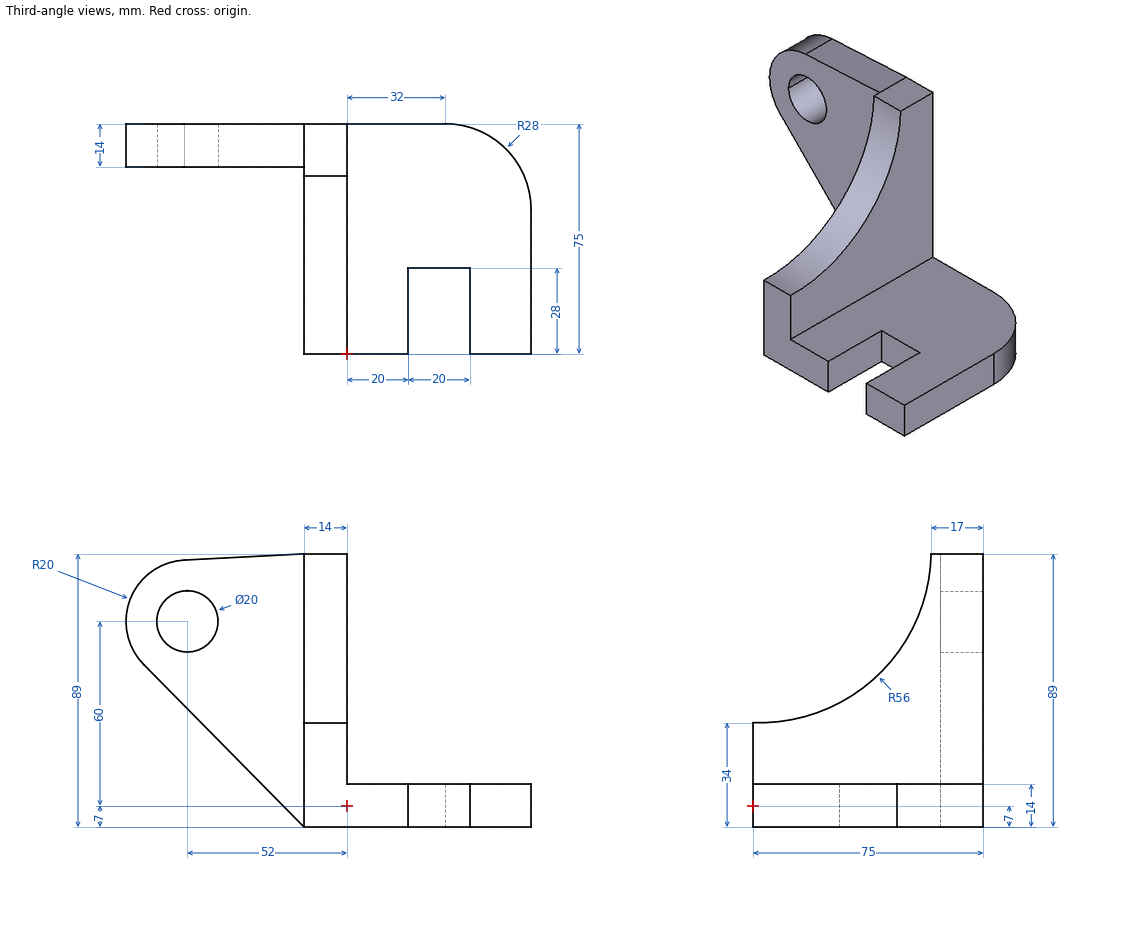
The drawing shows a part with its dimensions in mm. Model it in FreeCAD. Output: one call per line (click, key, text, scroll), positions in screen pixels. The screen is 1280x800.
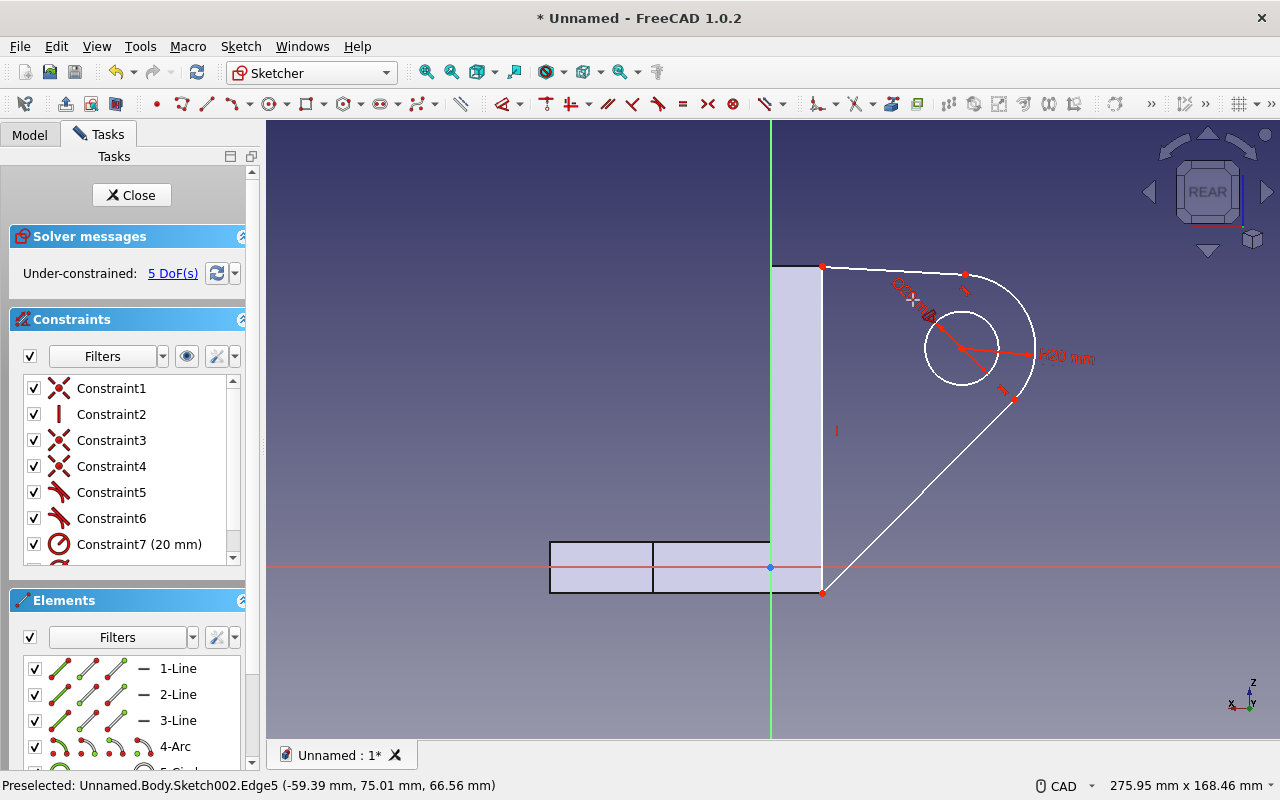
click(822, 365)
click(788, 430)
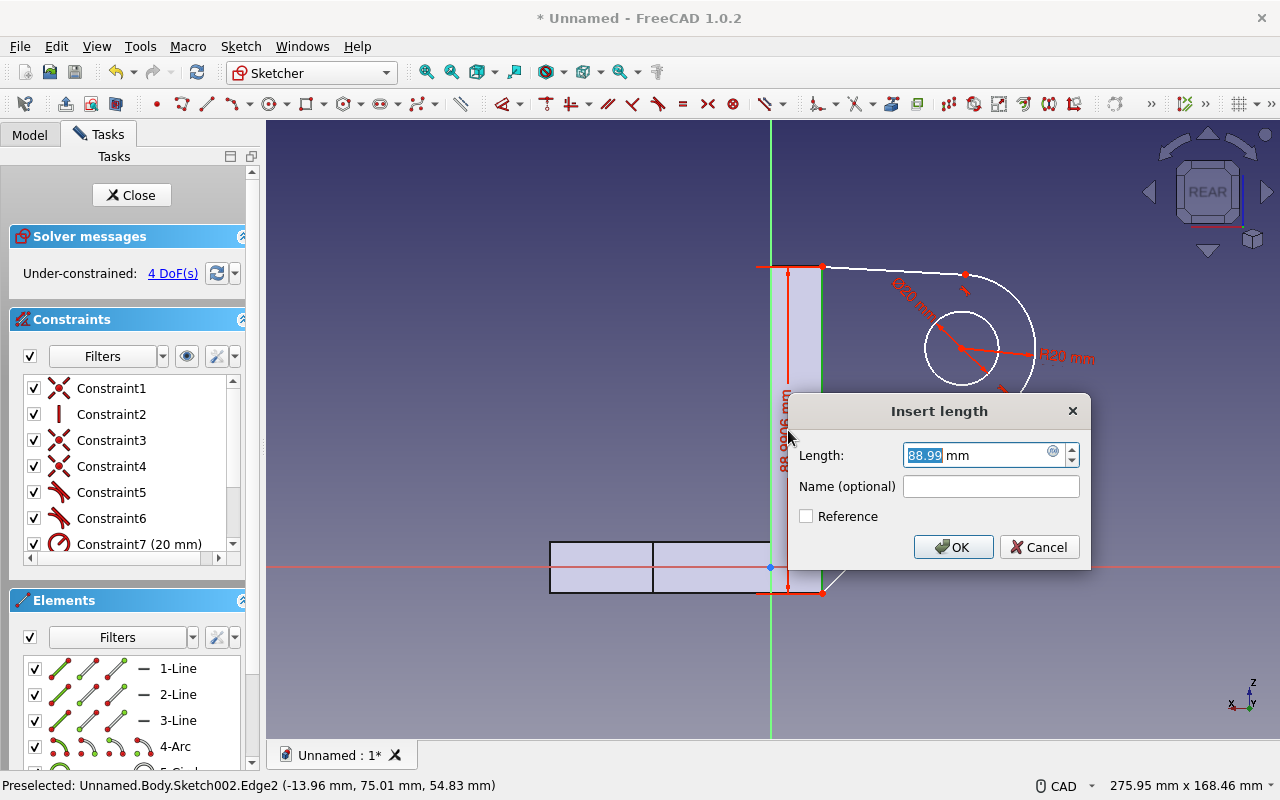
text(89)
key(Return)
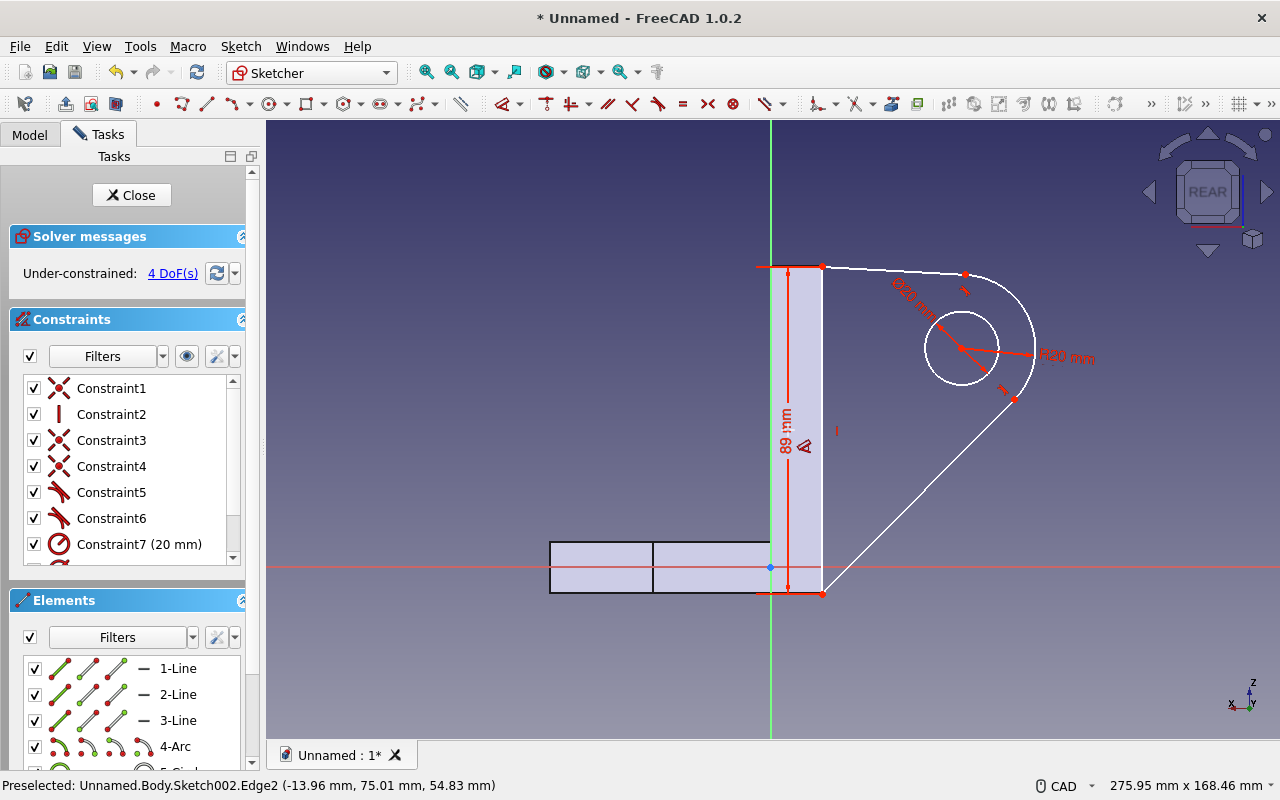
scroll(822, 594, up, 3)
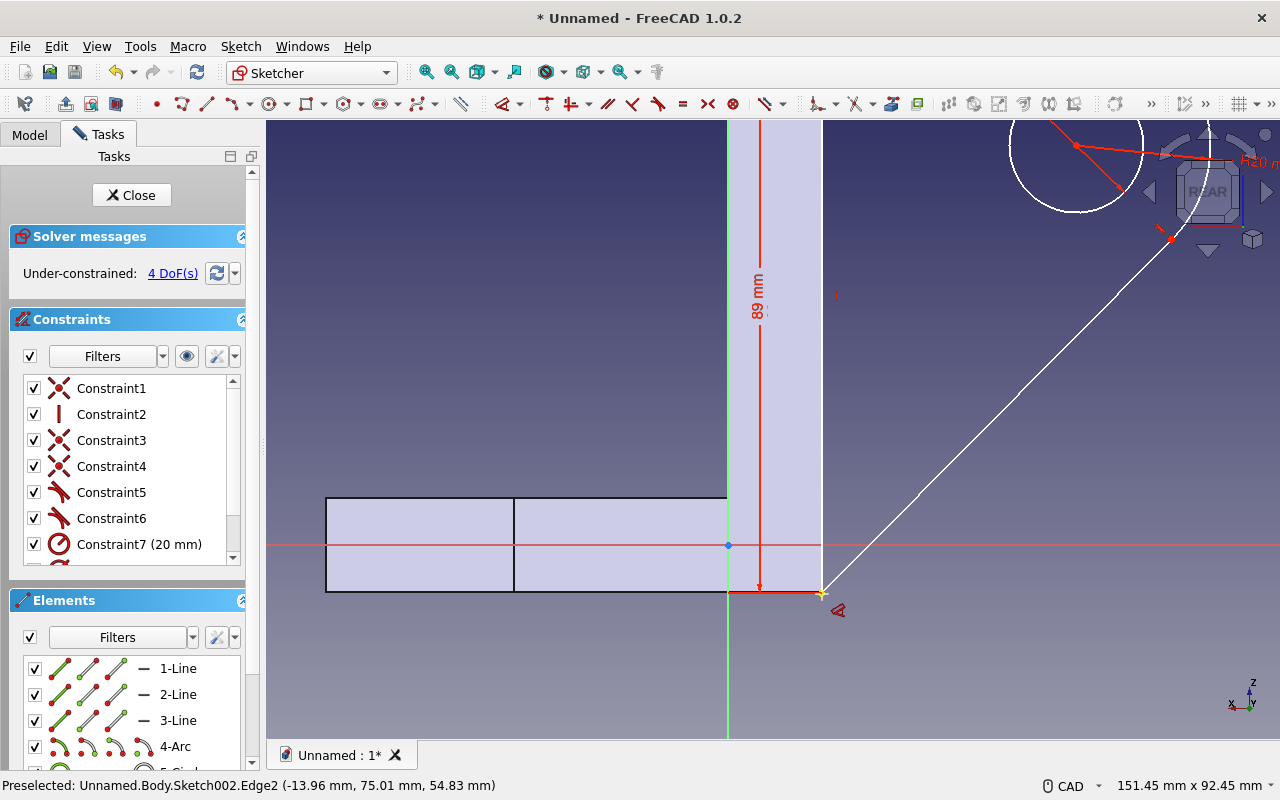
click(822, 593)
click(694, 569)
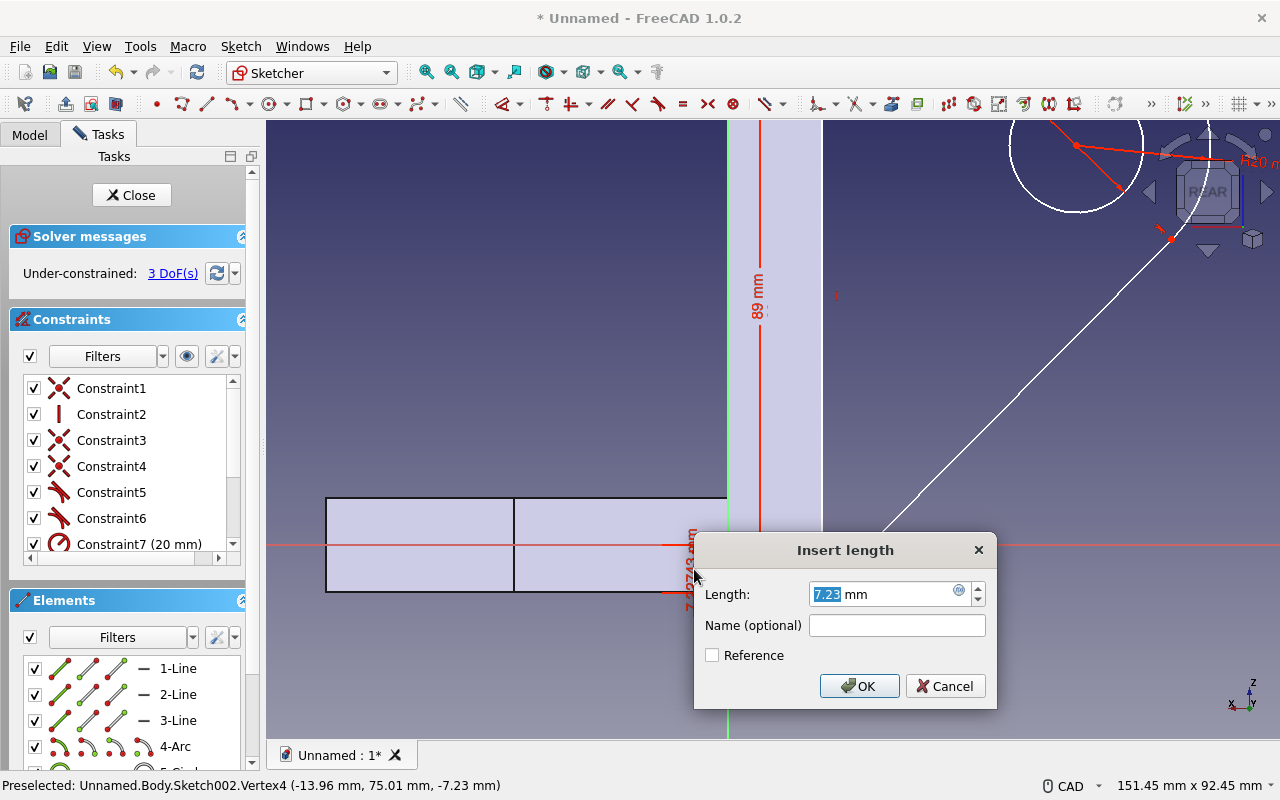
text(7)
key(Return)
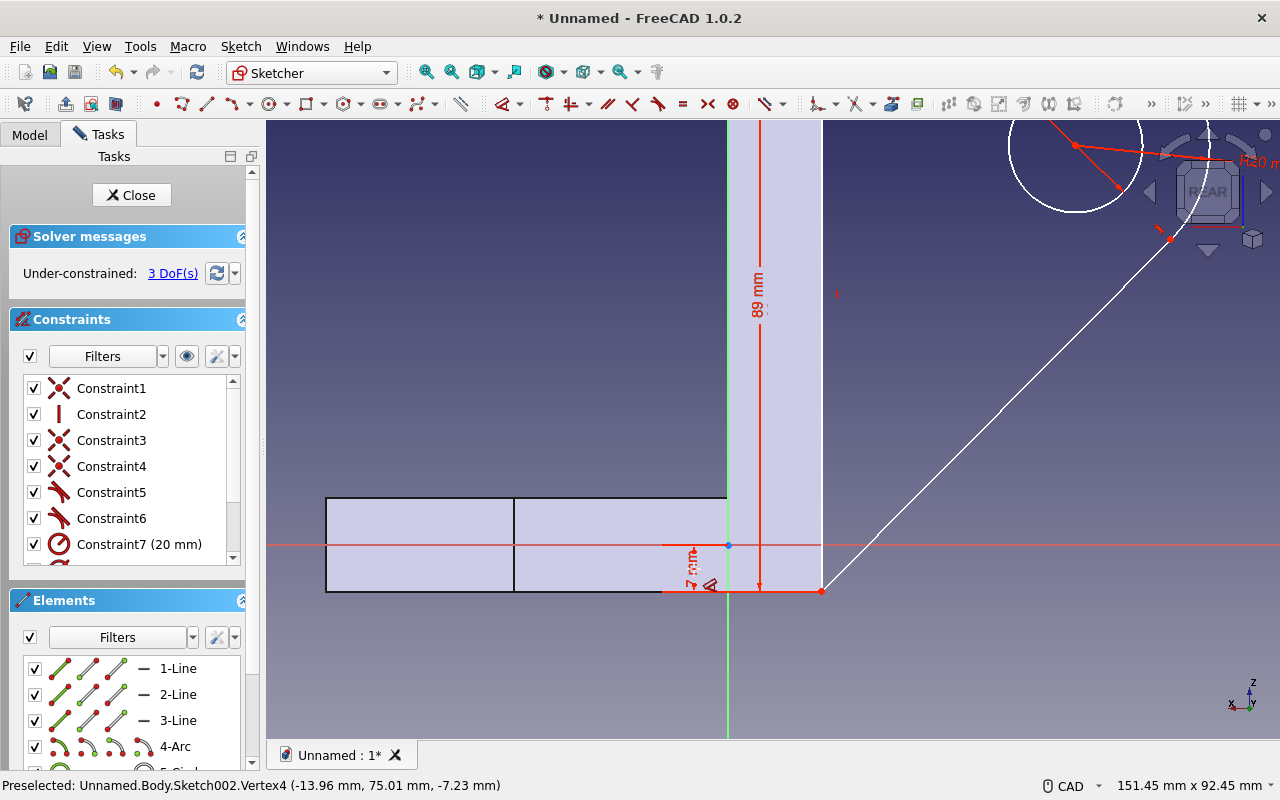
scroll(294, 705, down, 2)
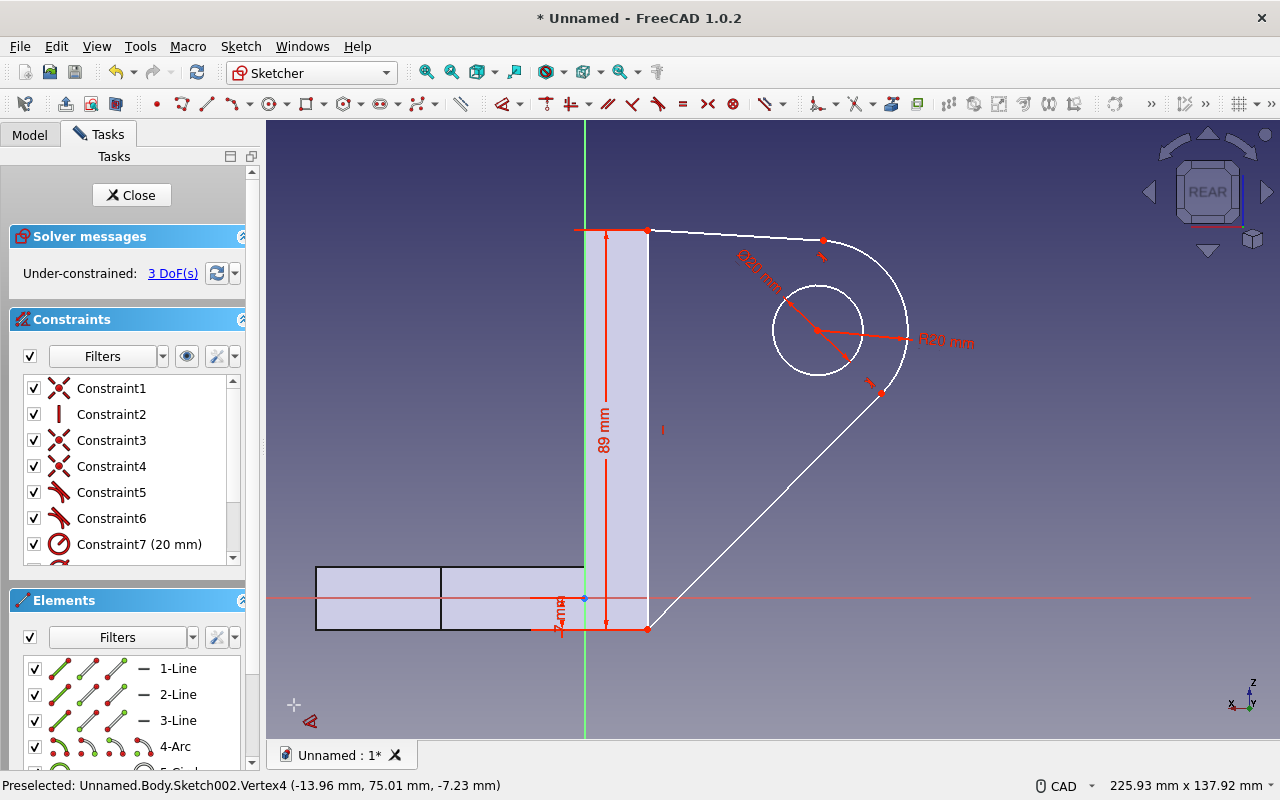
click(818, 330)
click(701, 632)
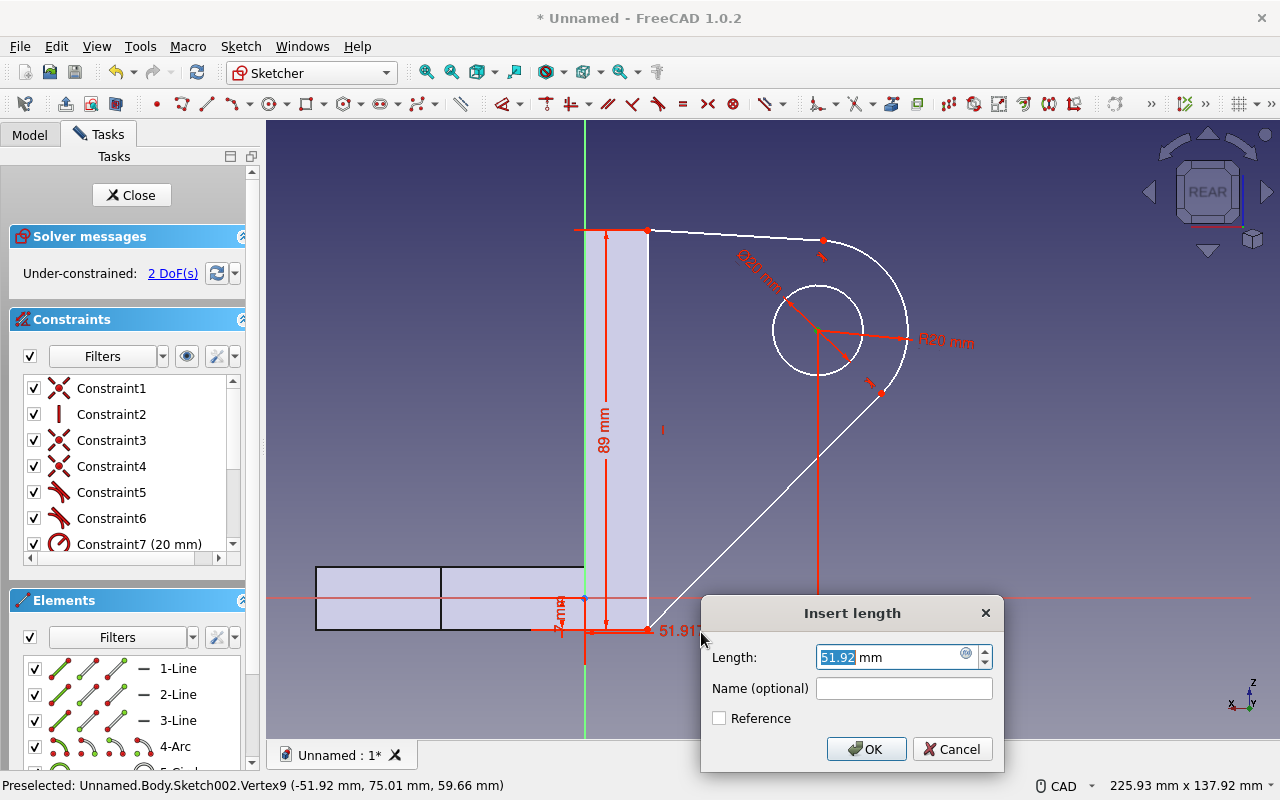
text(52)
key(Return)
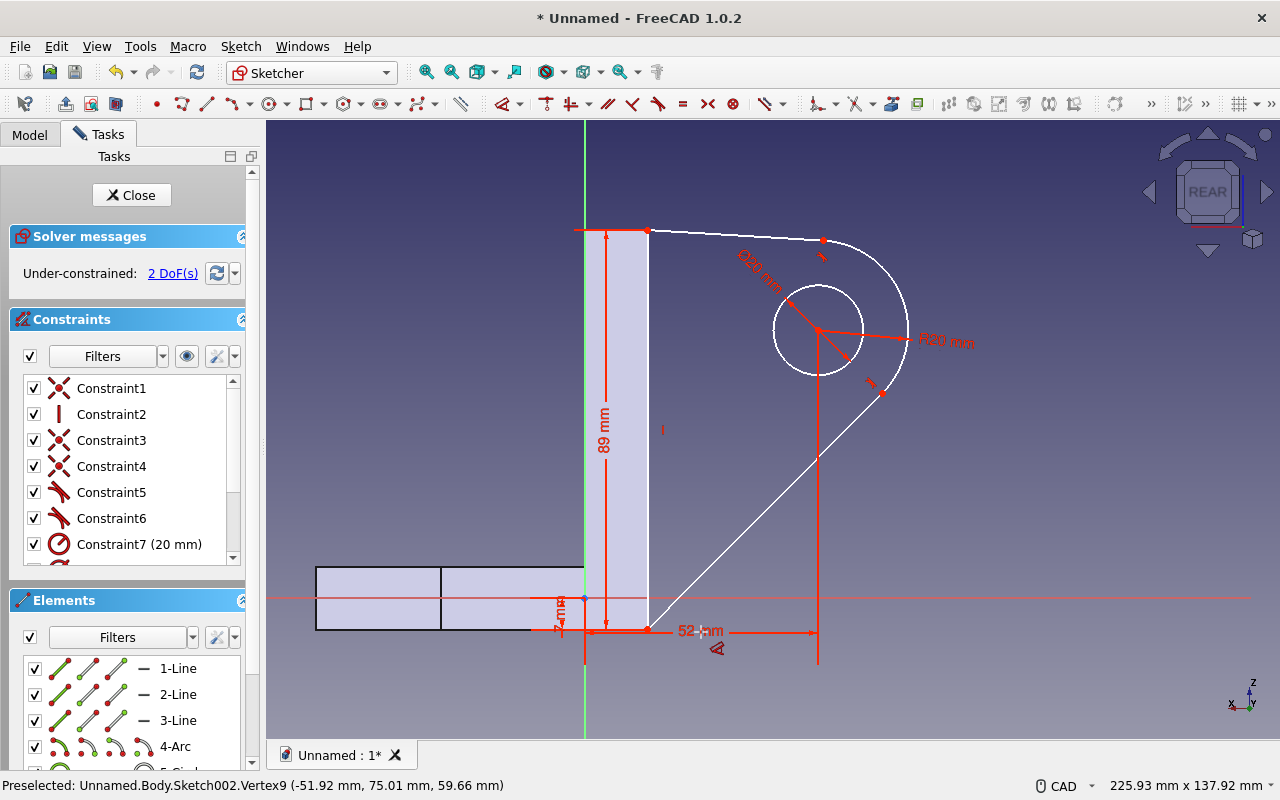
click(818, 330)
click(551, 464)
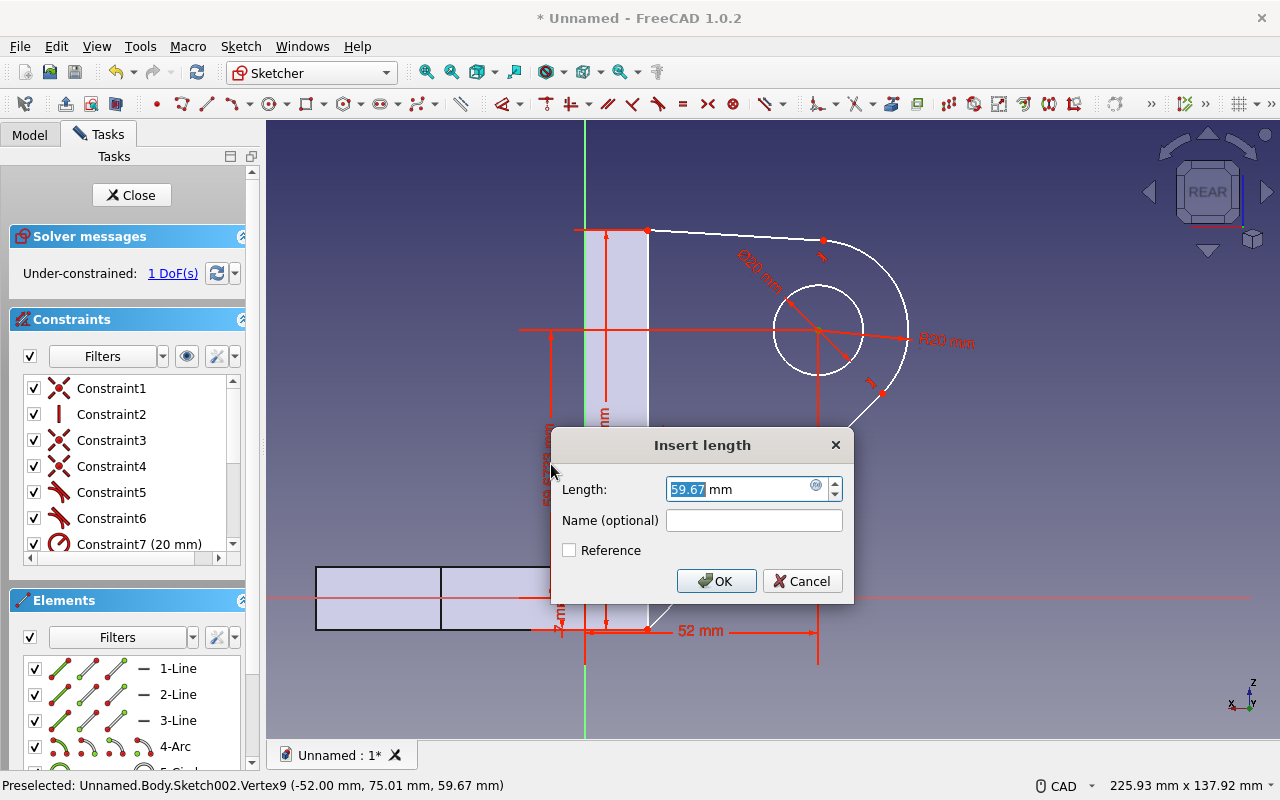
text(60)
key(Return)